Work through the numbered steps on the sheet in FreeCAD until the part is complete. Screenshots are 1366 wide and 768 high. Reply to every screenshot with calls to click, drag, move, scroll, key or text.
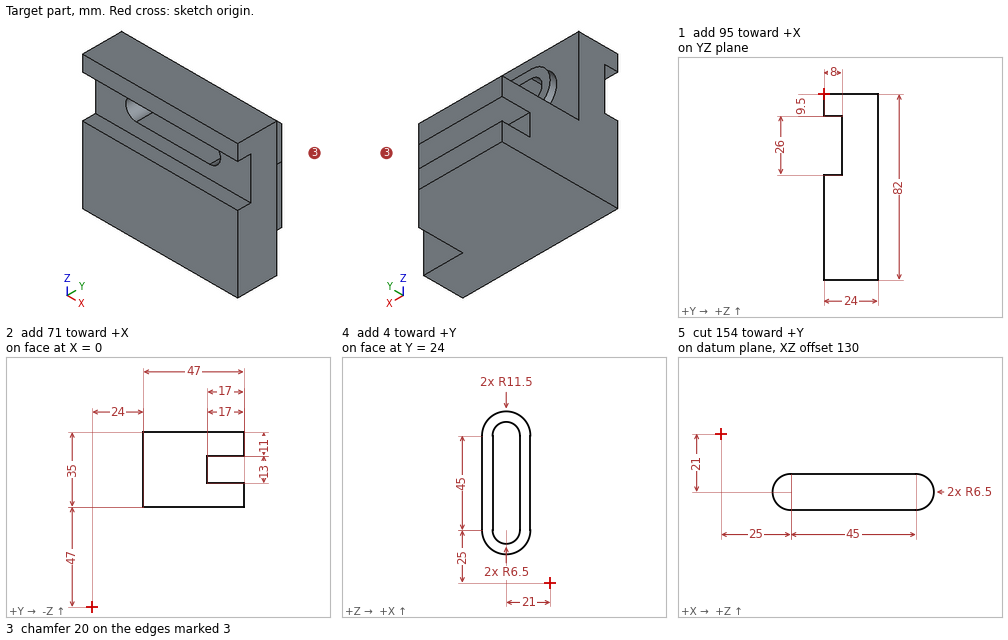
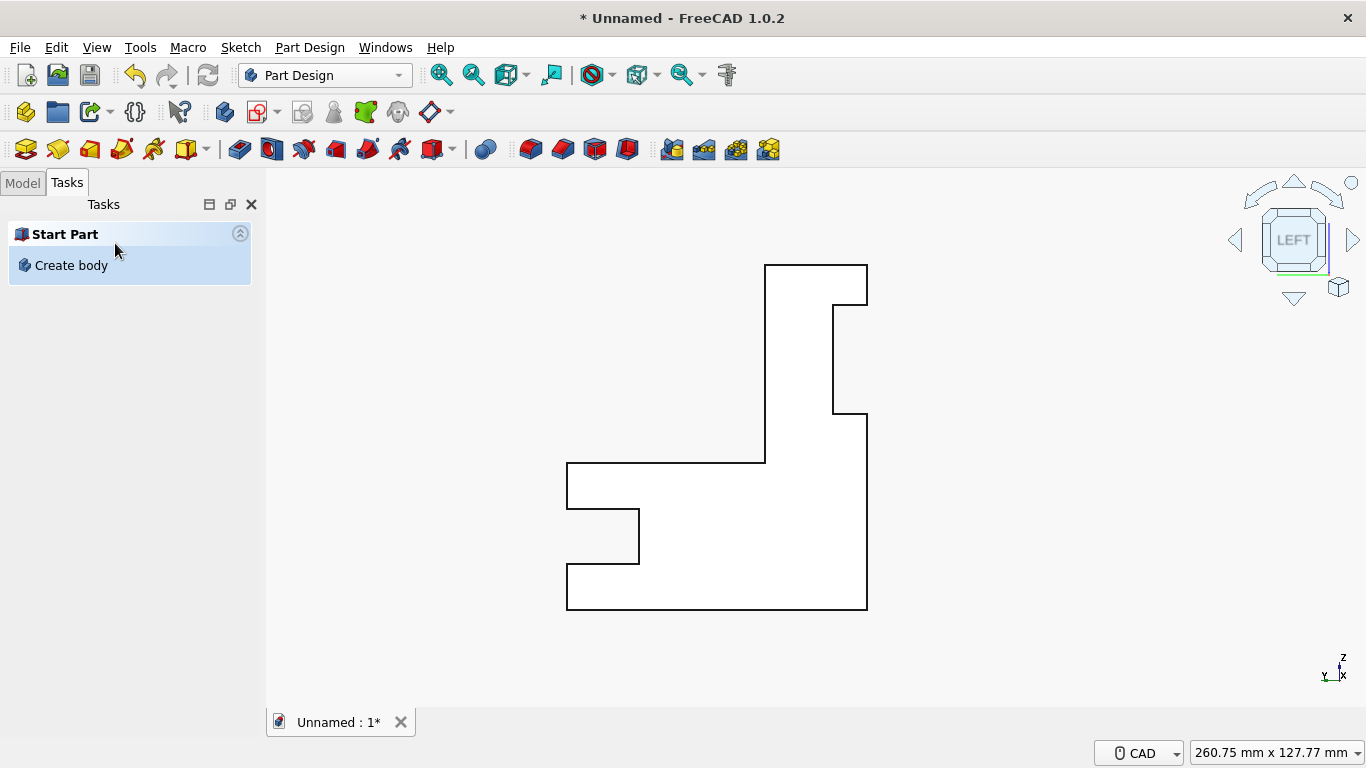
key(0)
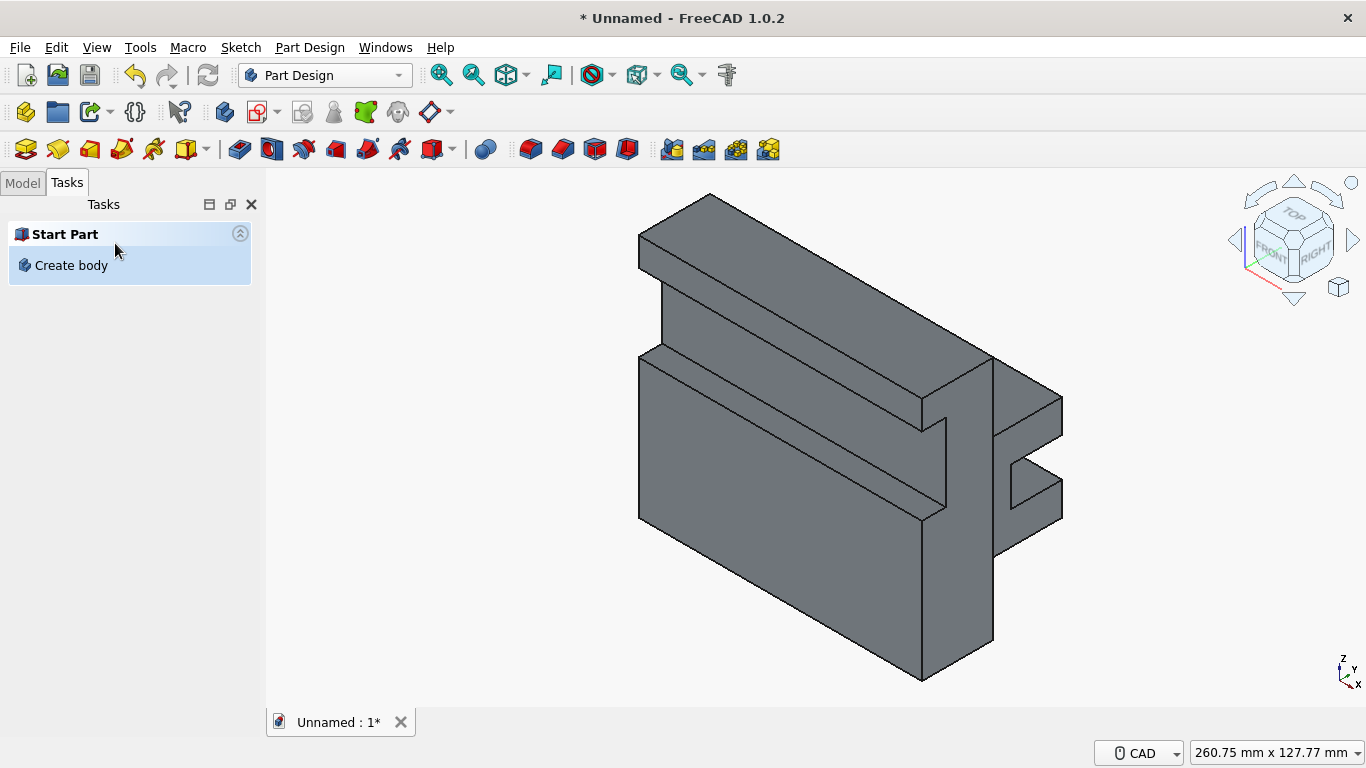
click(442, 76)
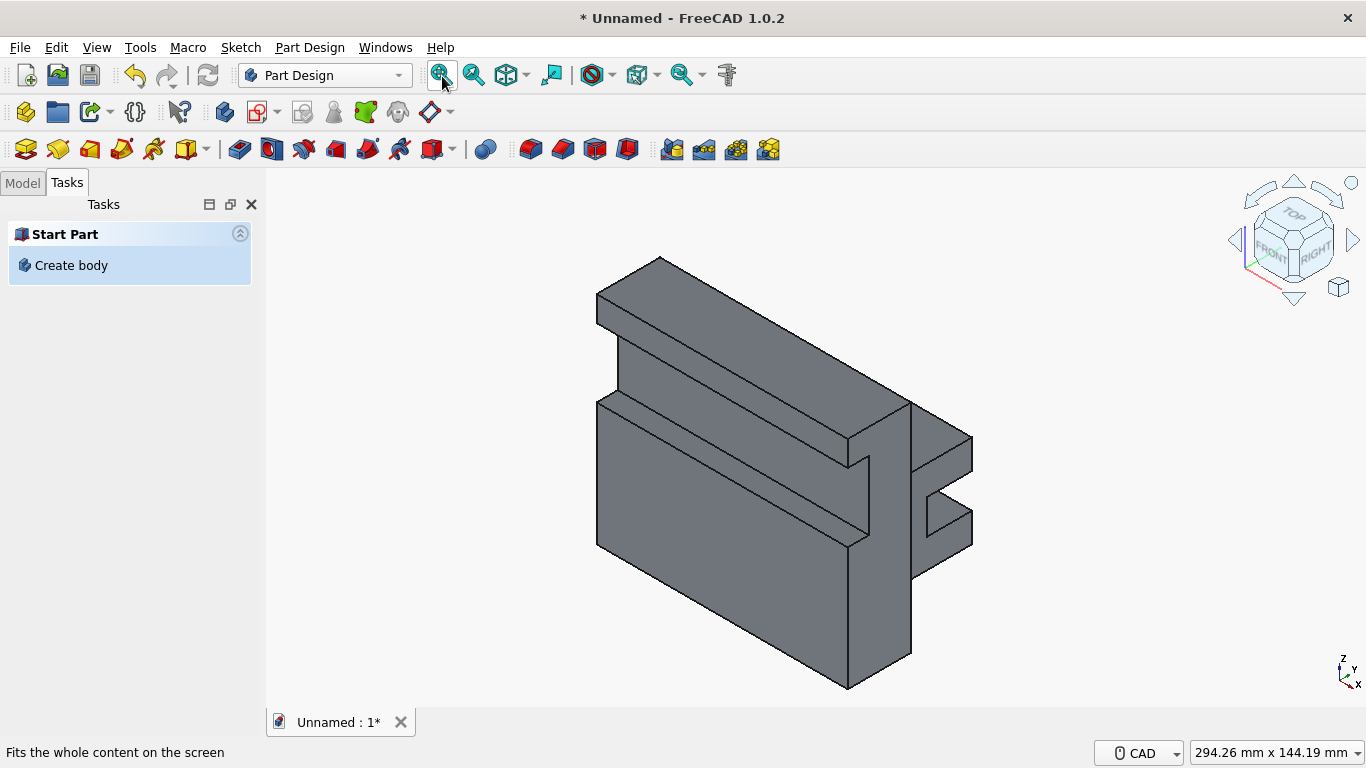
key(2)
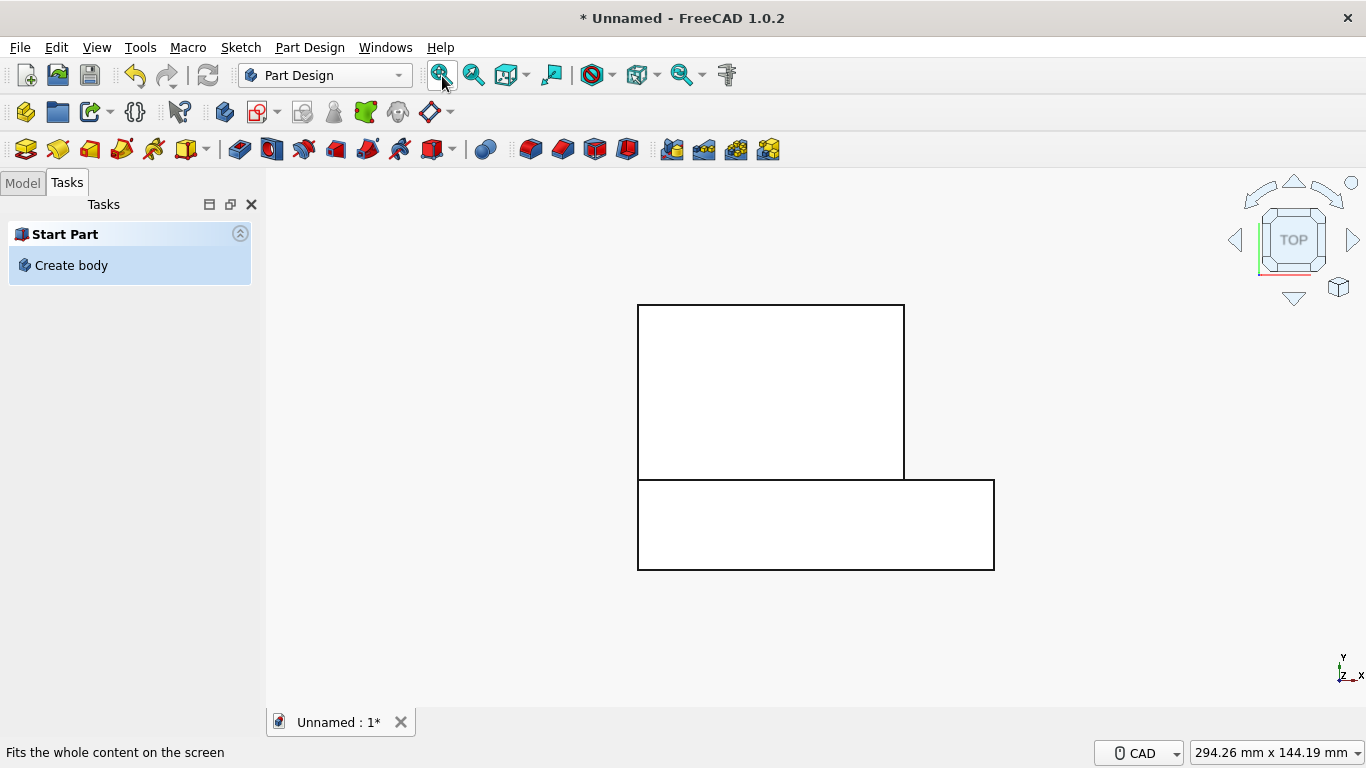
key(1)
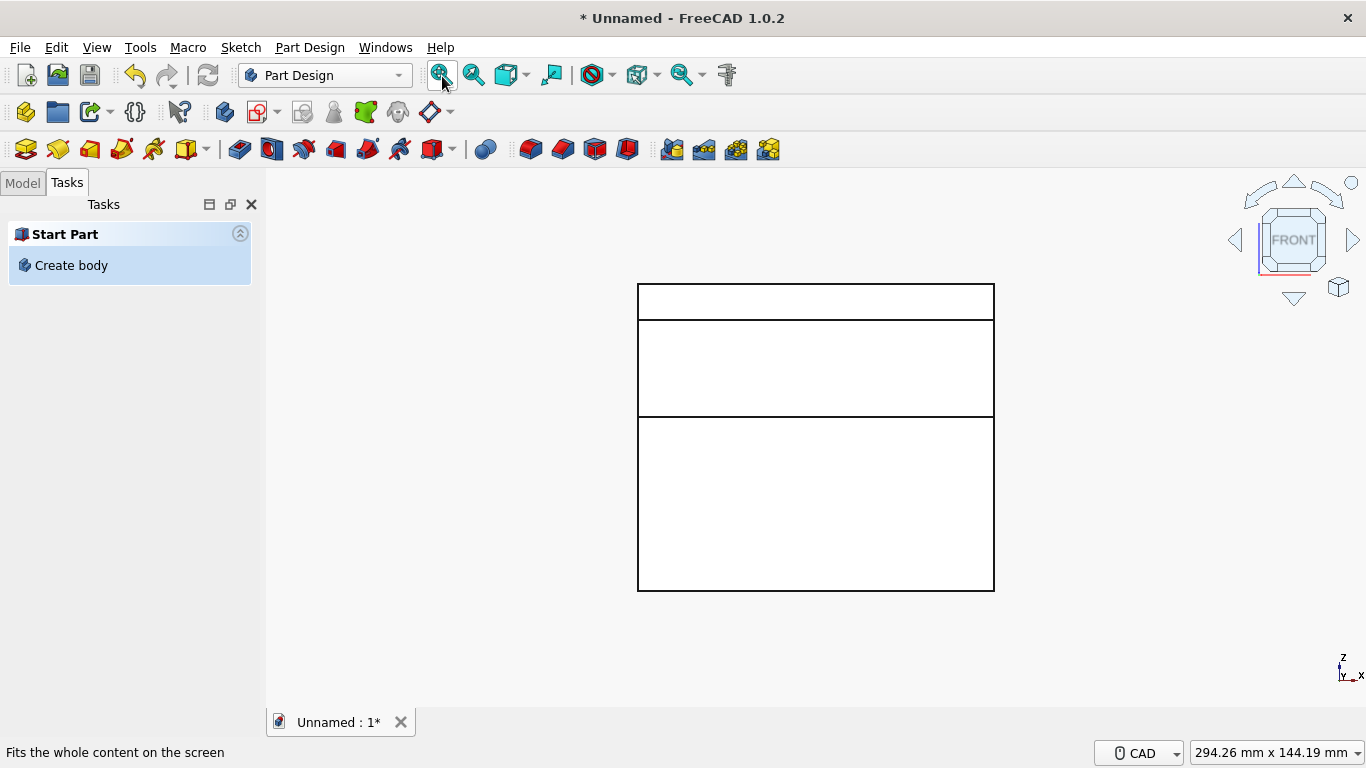
key(3)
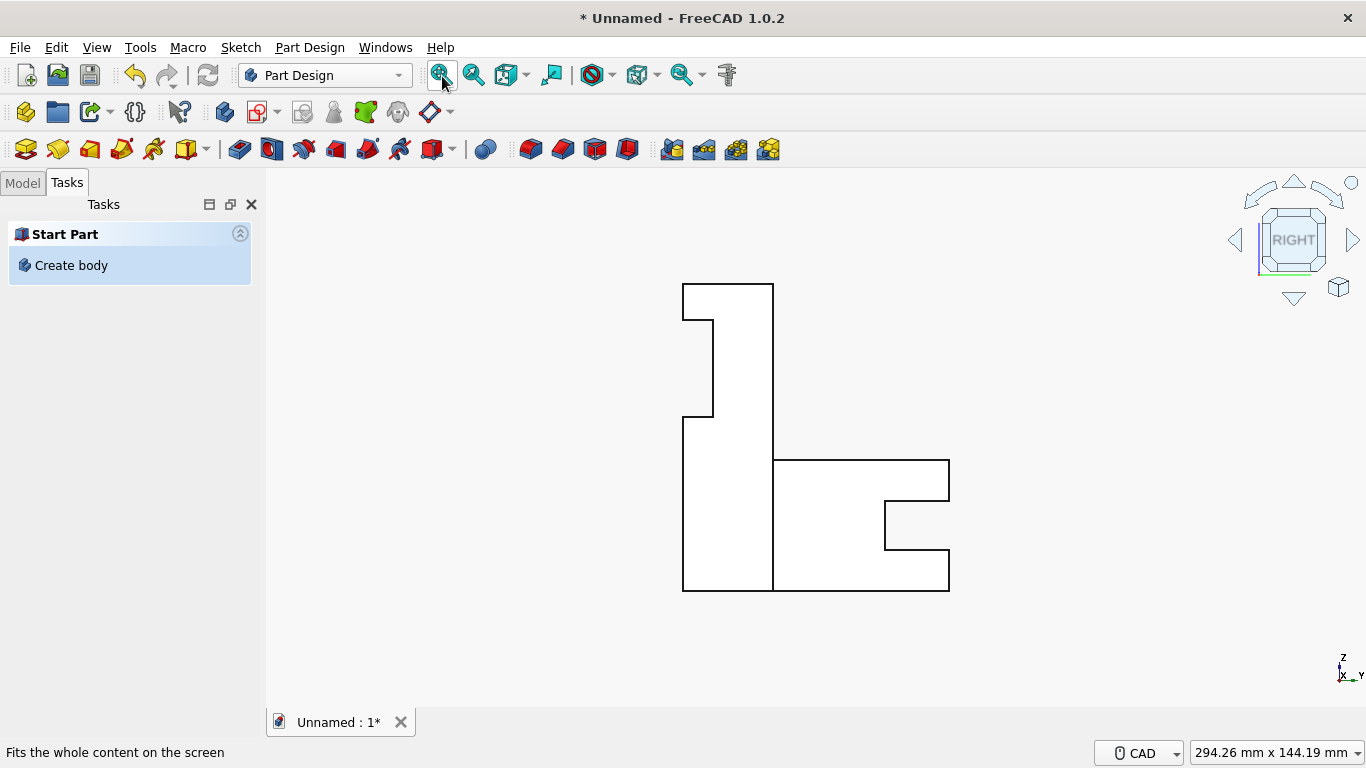
click(949, 479)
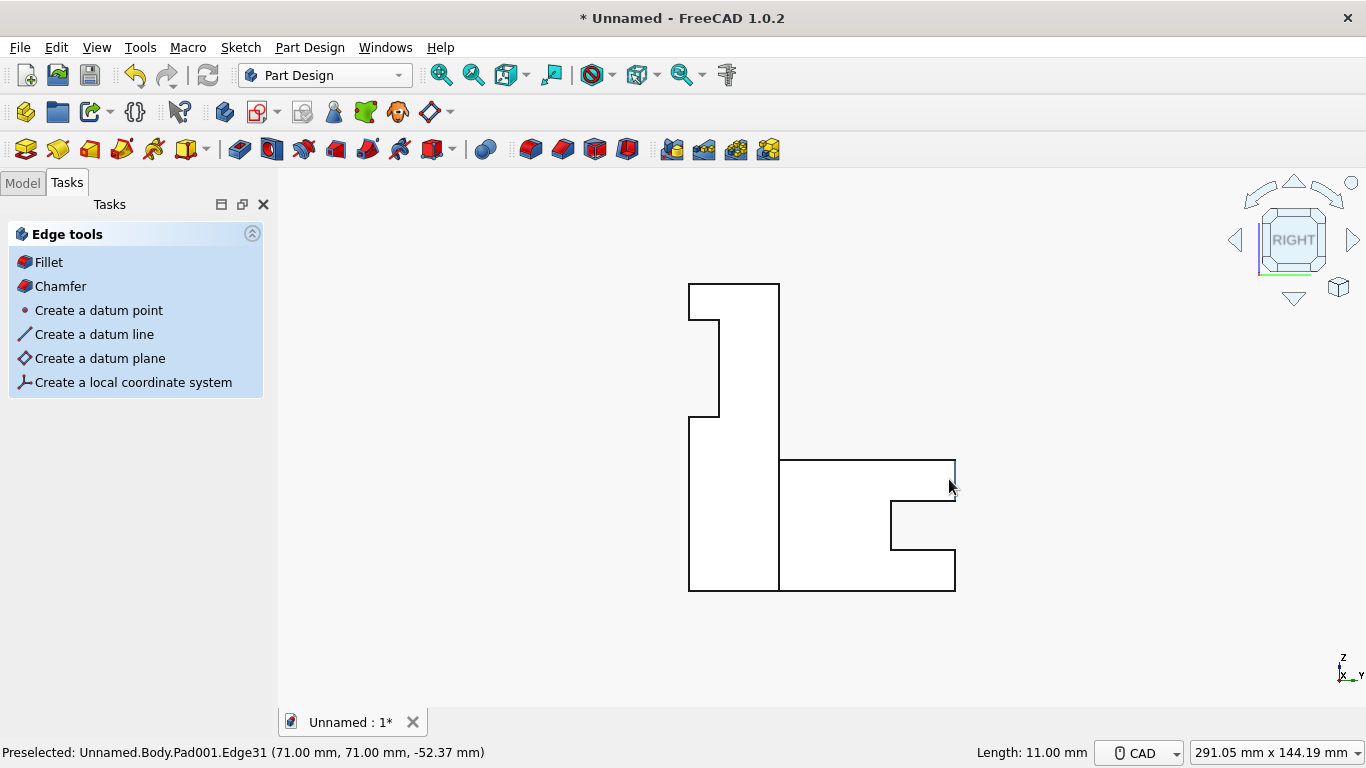
click(564, 150)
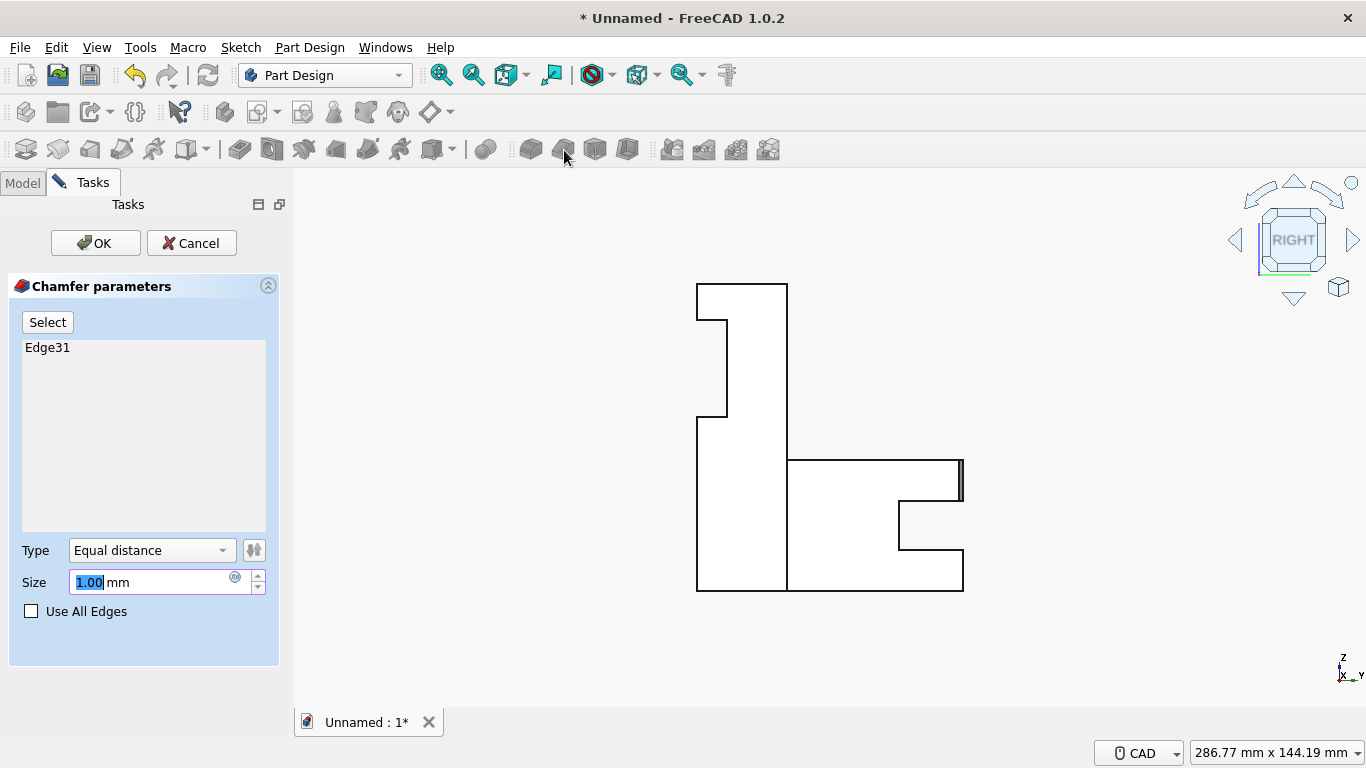
text(20)
key(Tab)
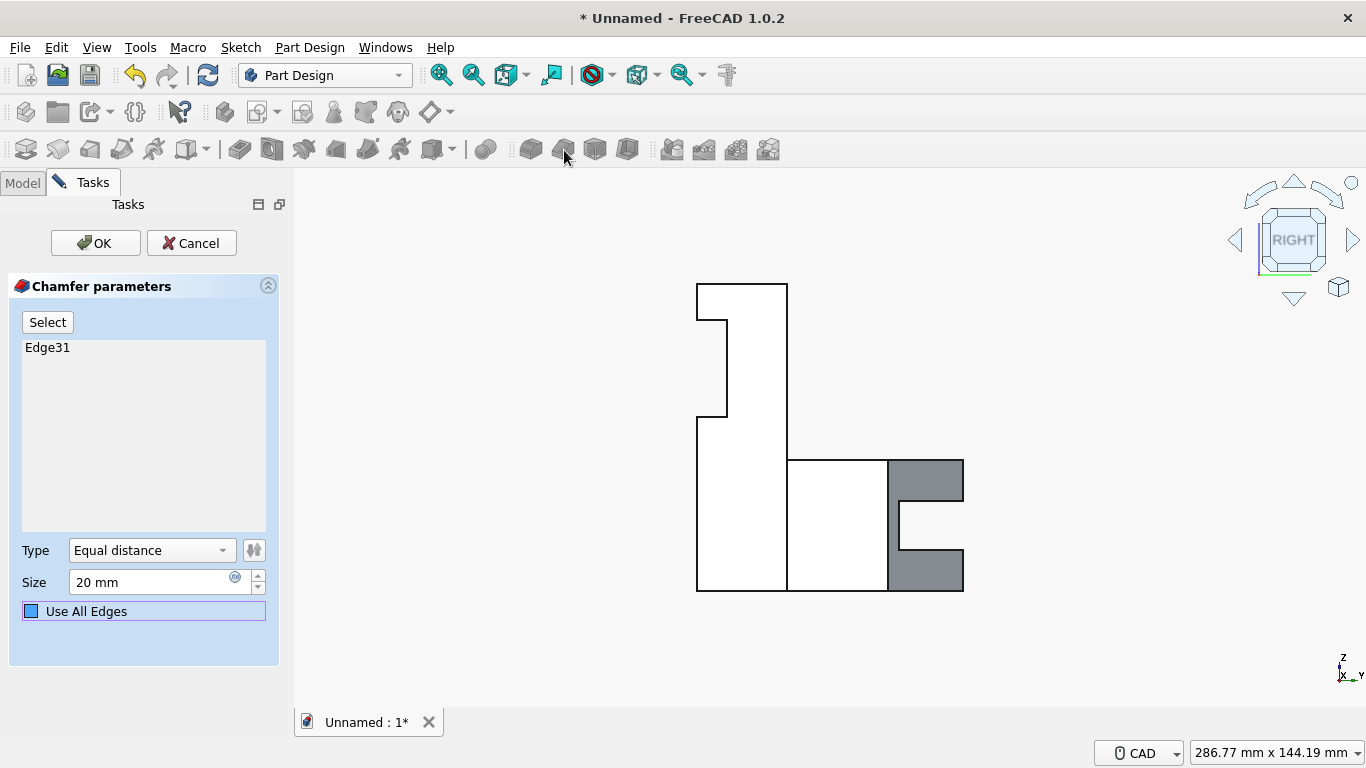
click(96, 243)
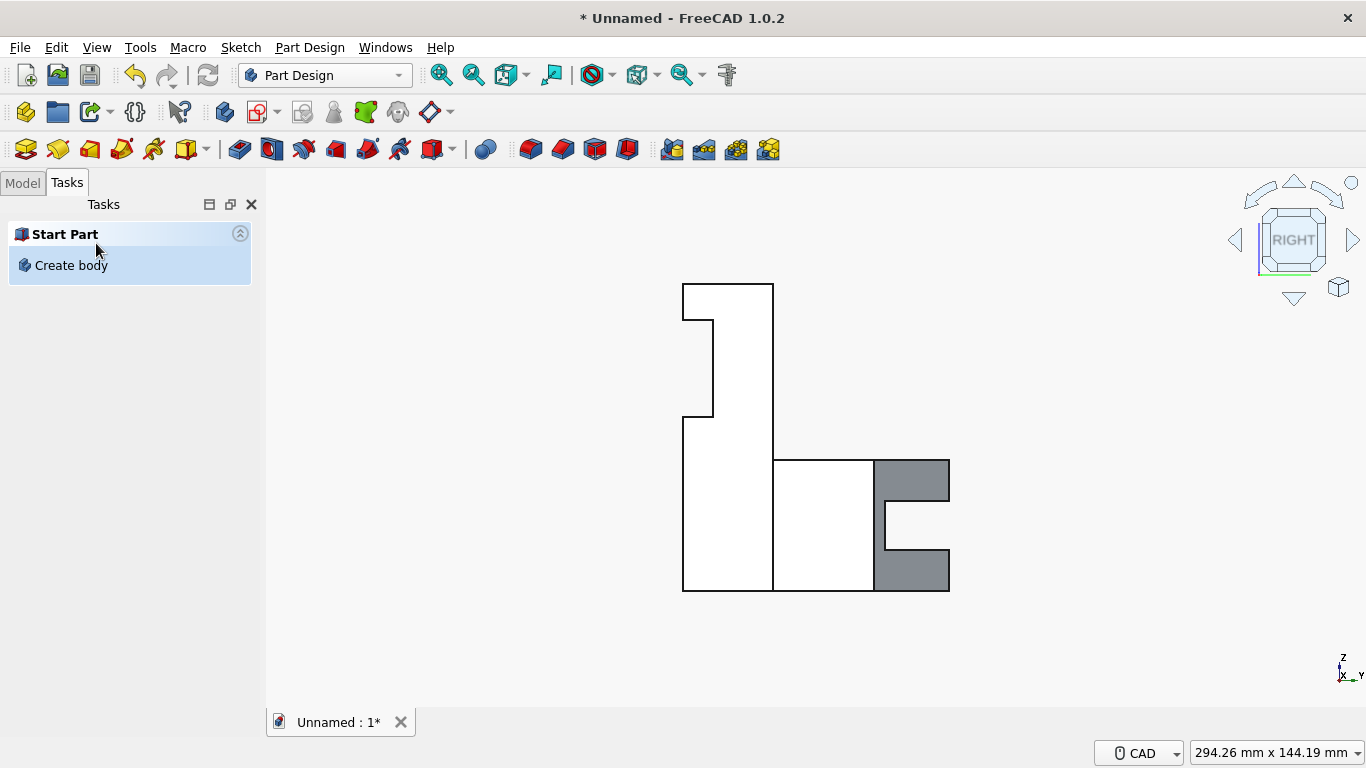
key(4)